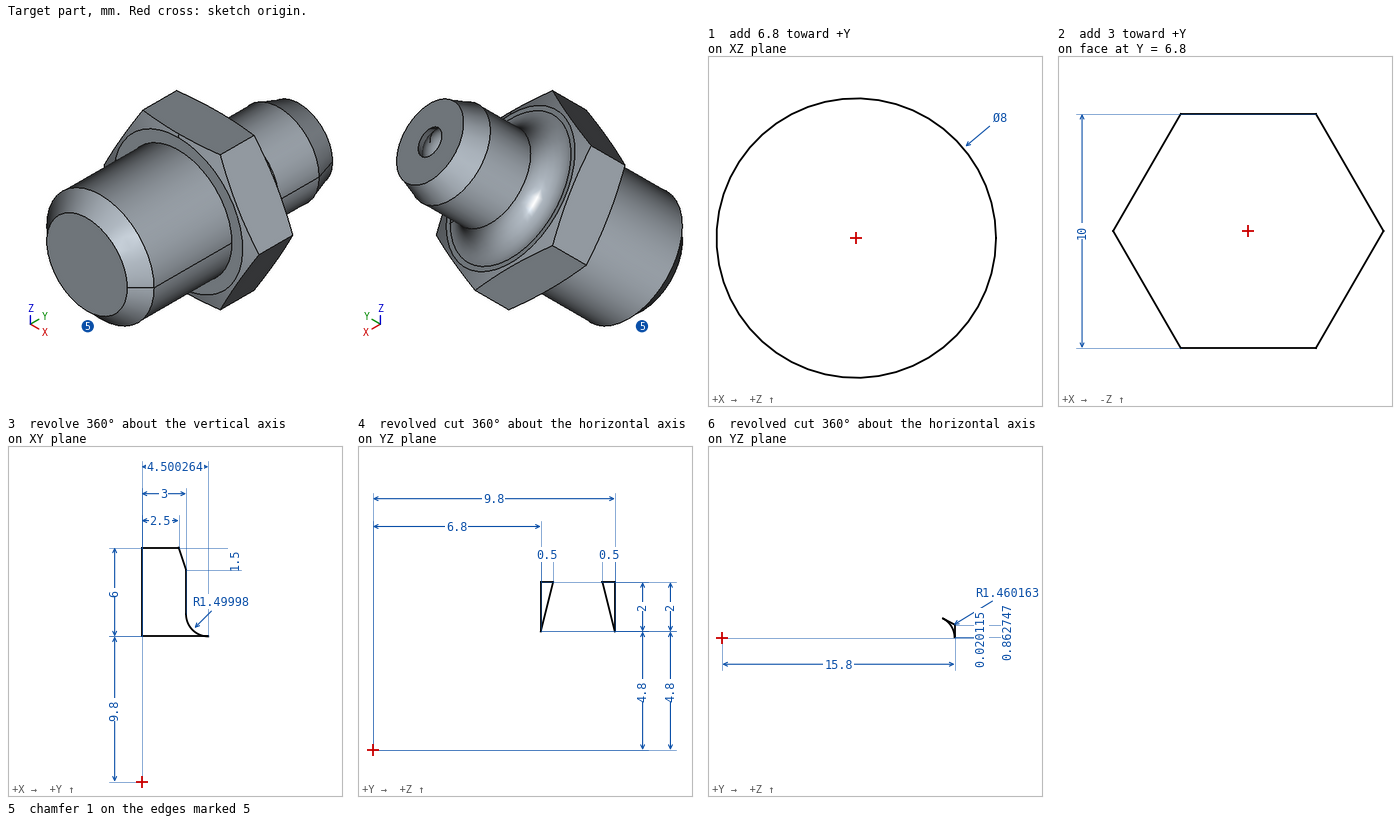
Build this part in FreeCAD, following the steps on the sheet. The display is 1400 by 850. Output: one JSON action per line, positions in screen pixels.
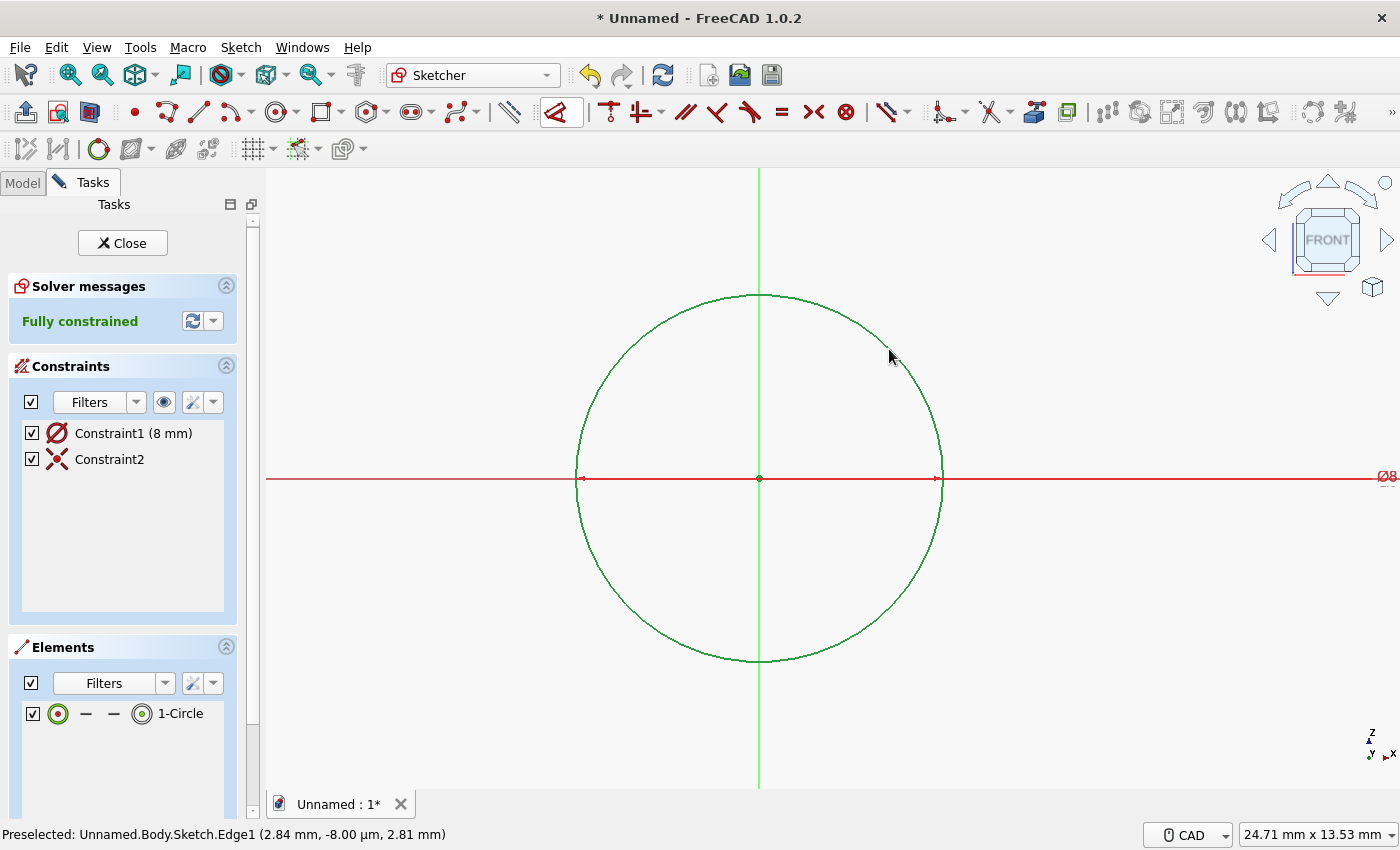
{"action": "left_click", "coordinate": [123, 243]}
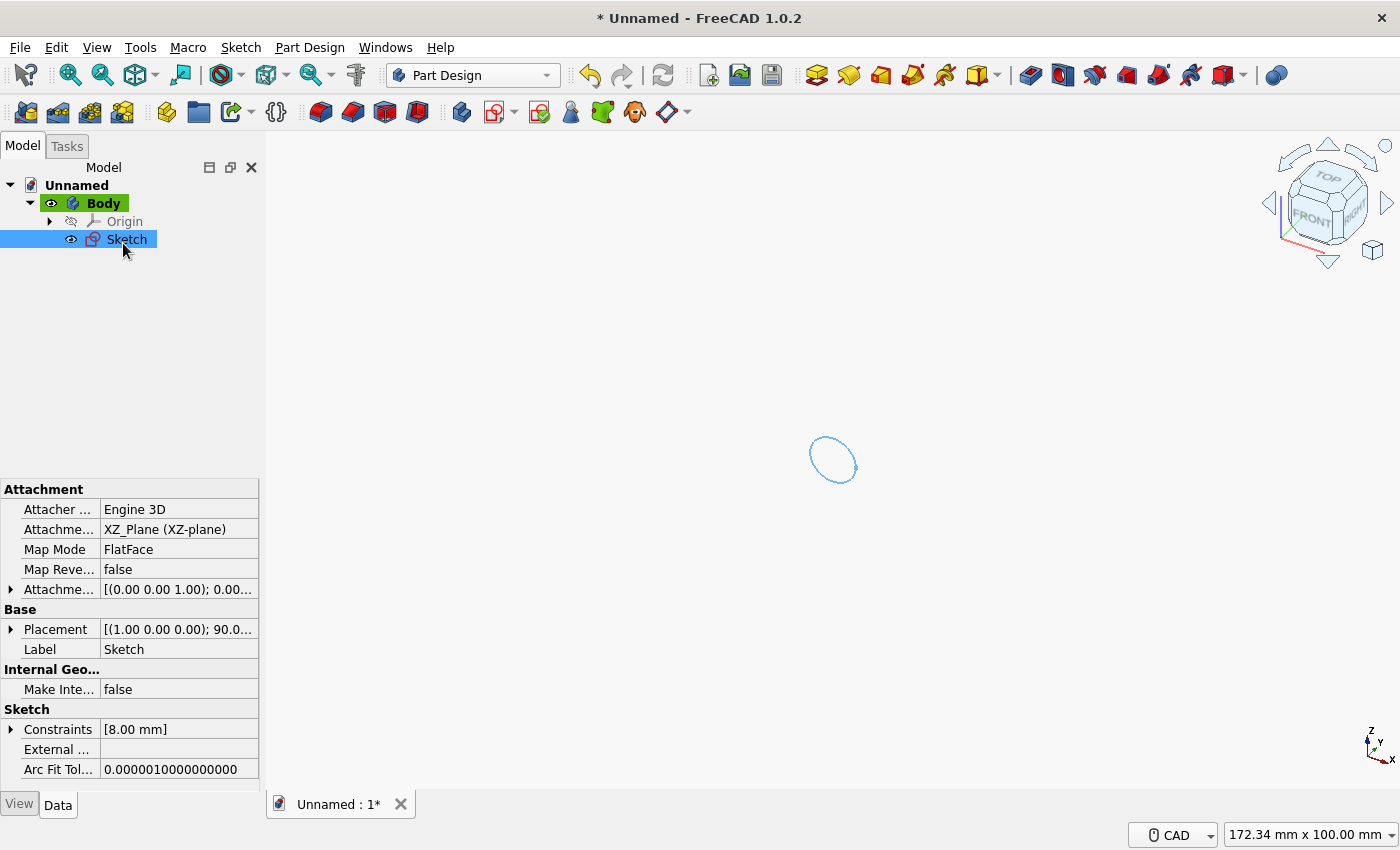
{"action": "left_click", "coordinate": [818, 76]}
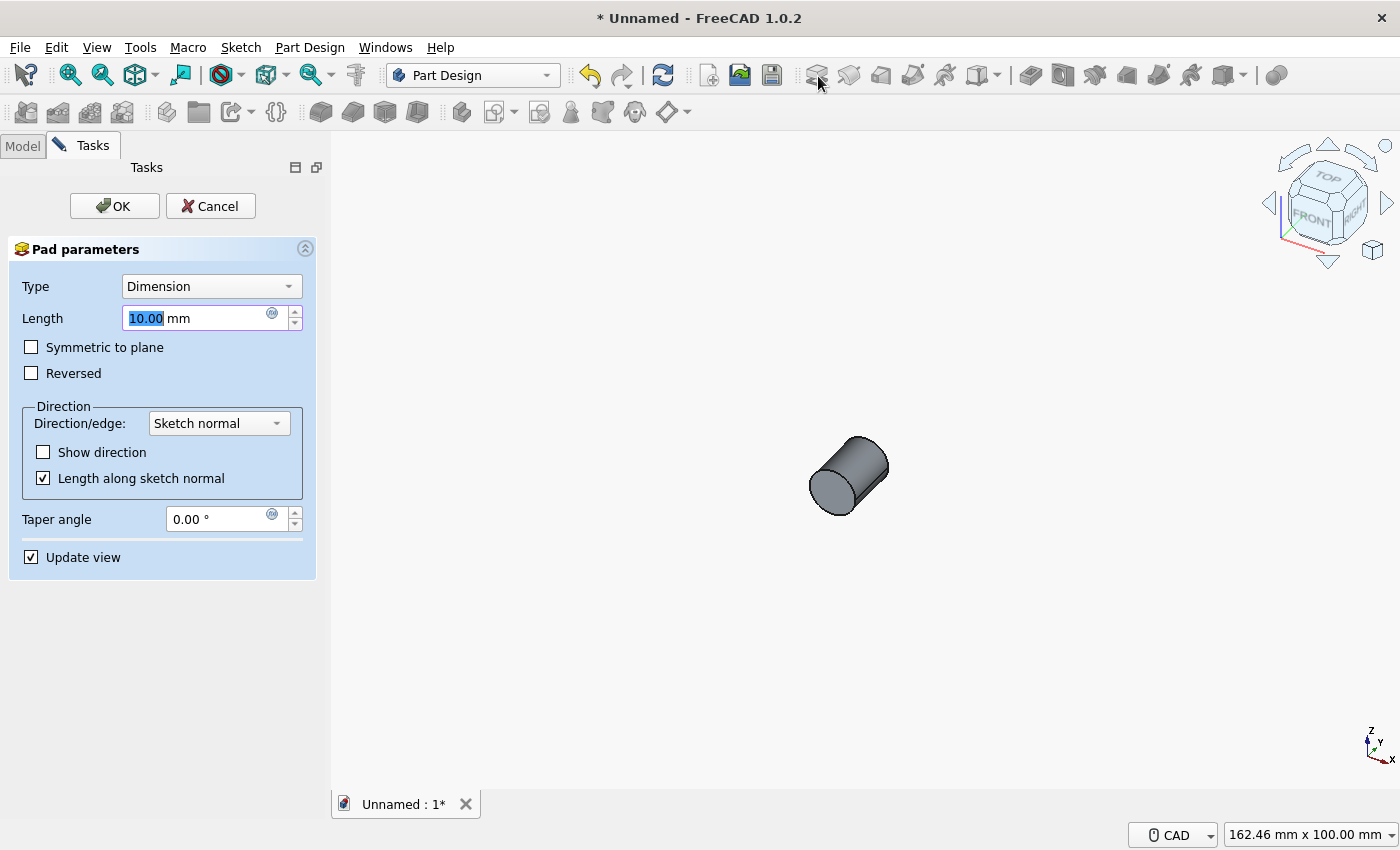
{"action": "type", "text": "6.8"}
{"action": "key", "text": "Tab"}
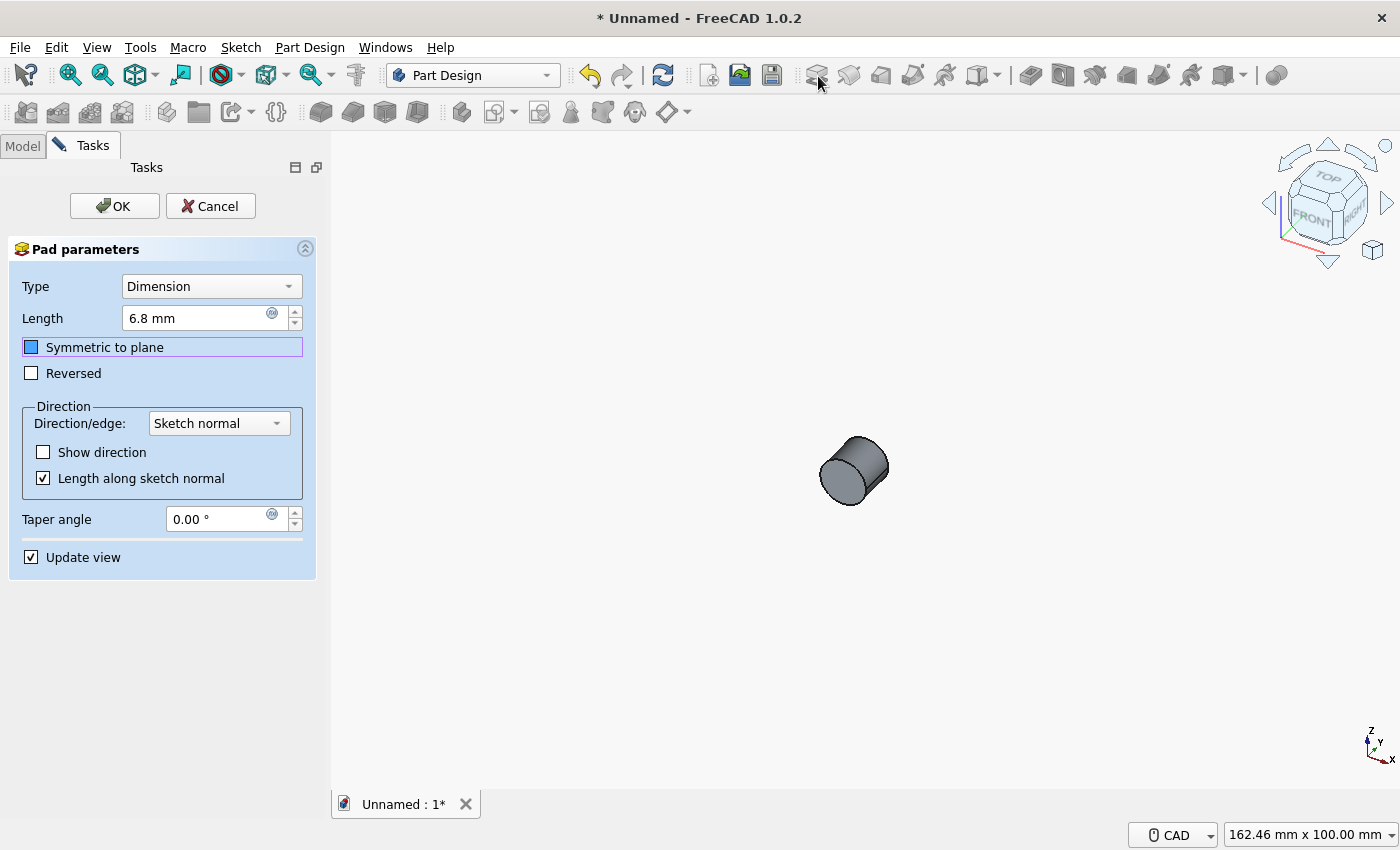
{"action": "left_click", "coordinate": [30, 373]}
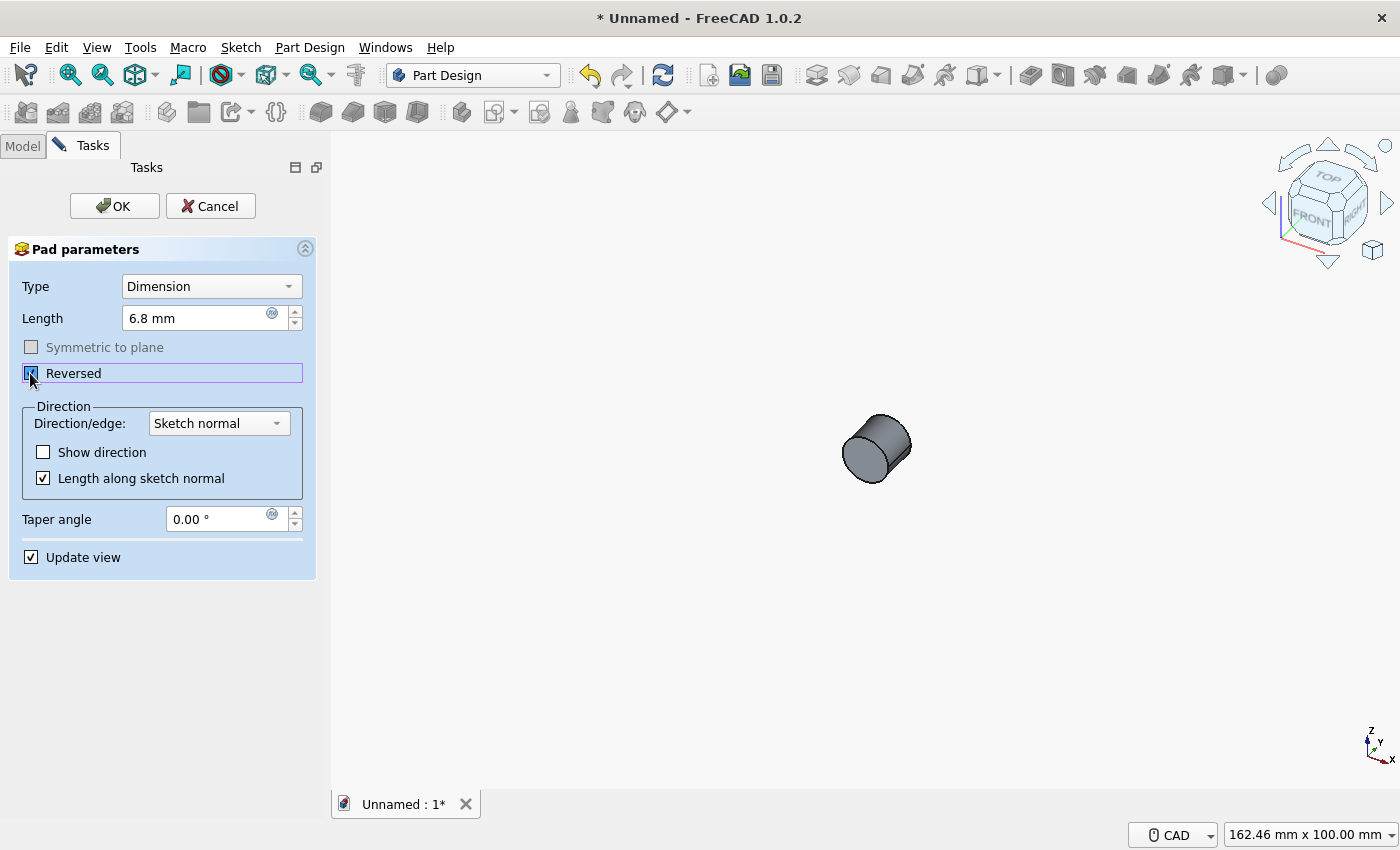
{"action": "left_click", "coordinate": [115, 206]}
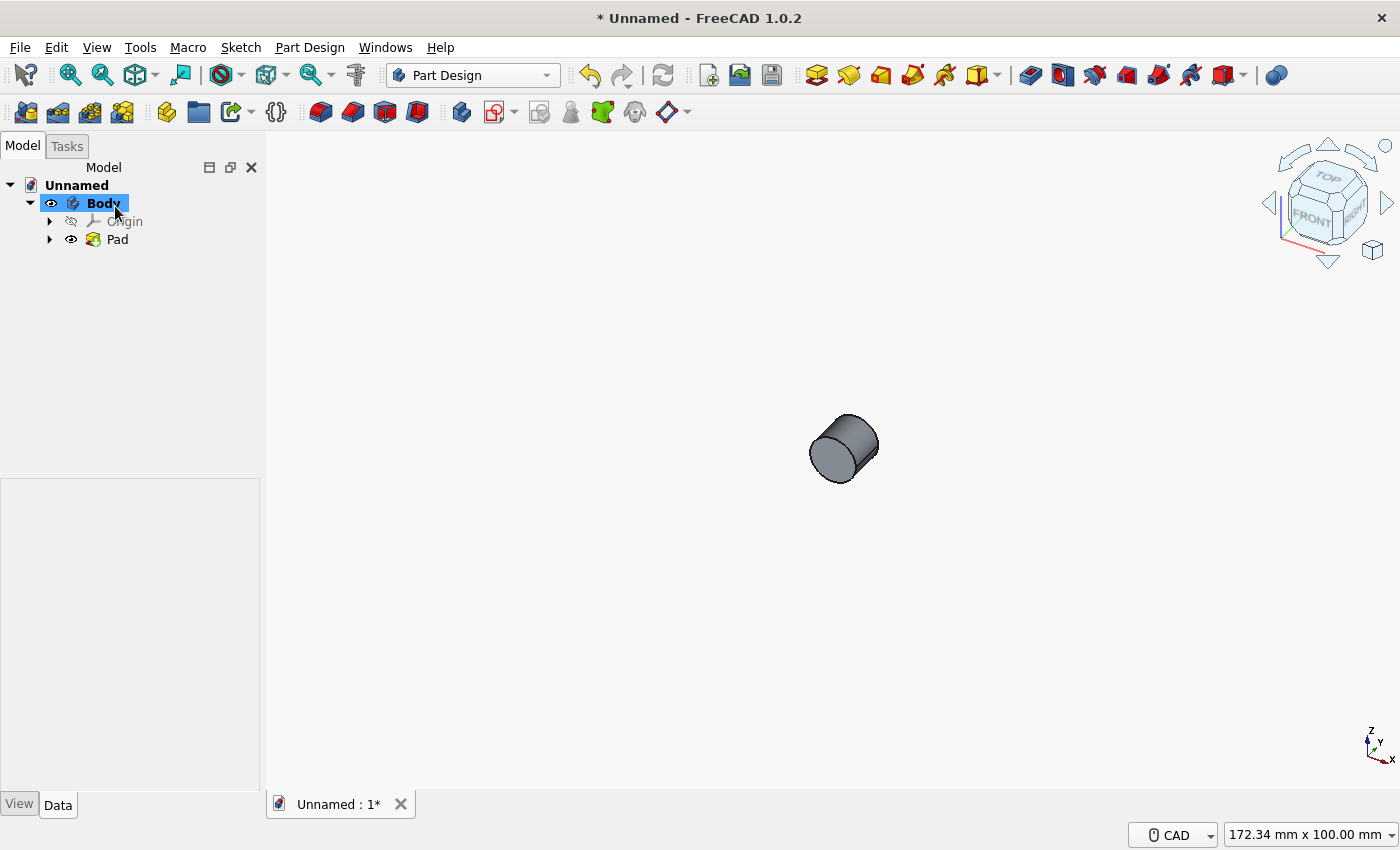
{"action": "left_click", "coordinate": [72, 76]}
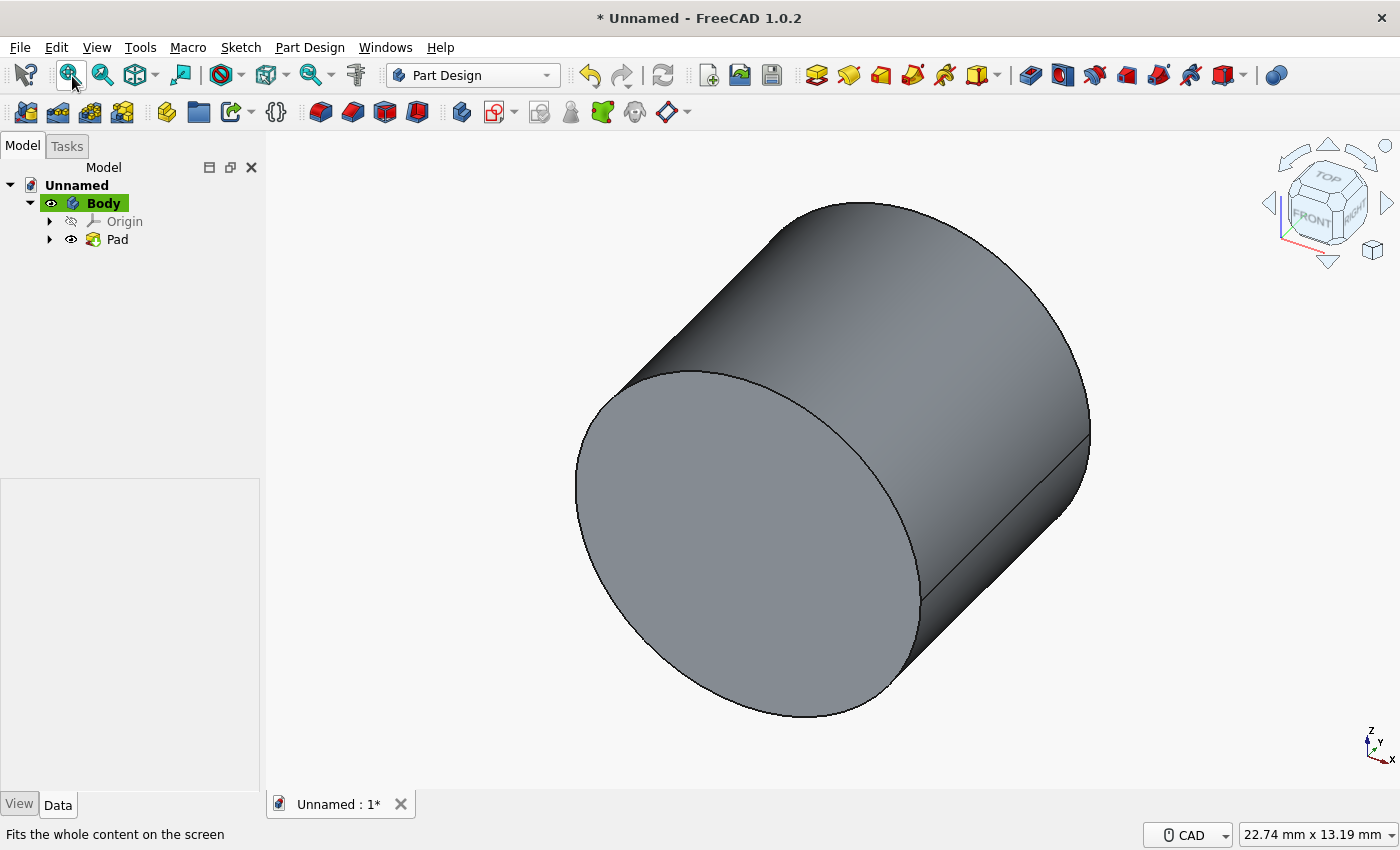
{"action": "key", "text": "4"}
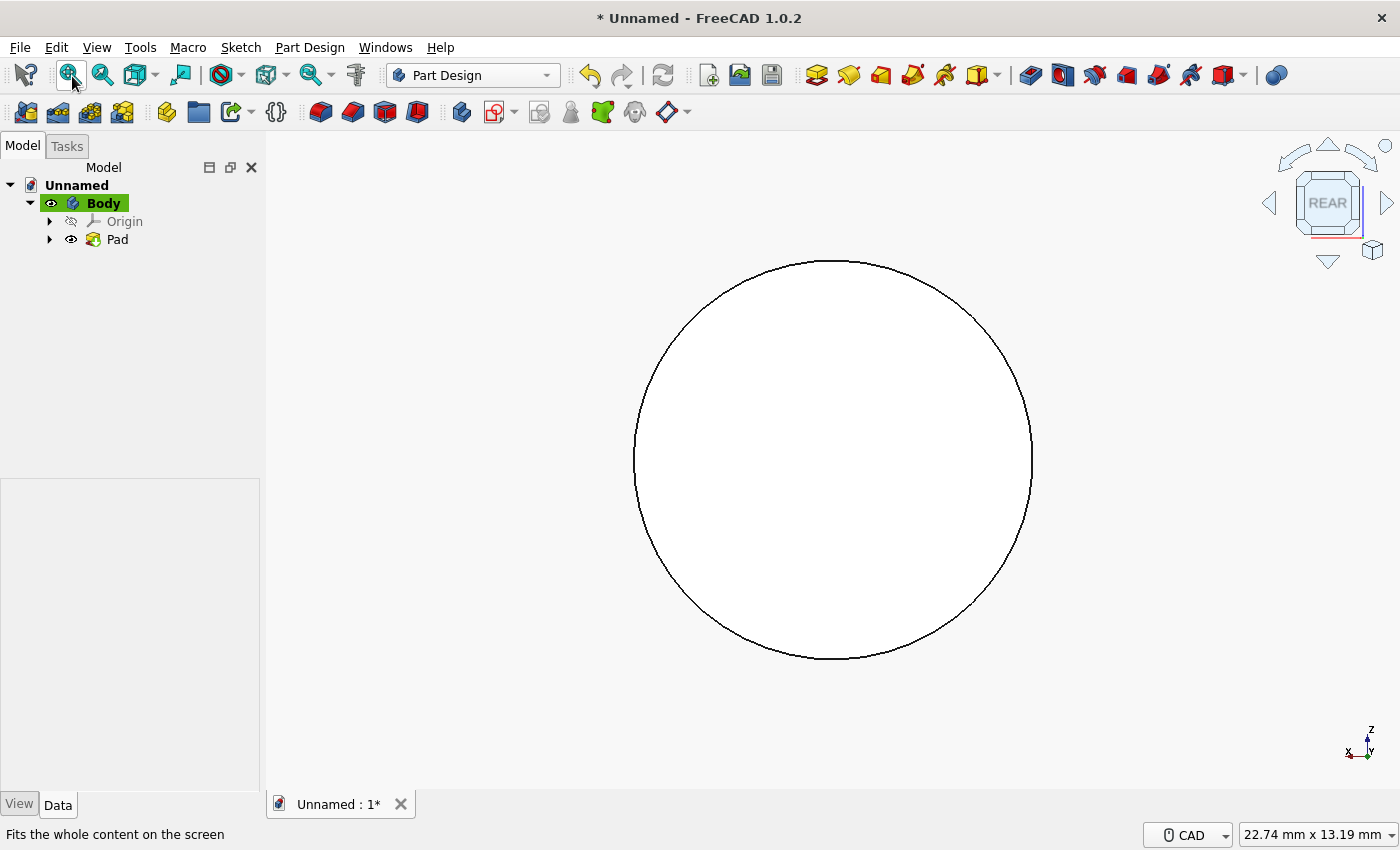
{"action": "left_click", "coordinate": [833, 459]}